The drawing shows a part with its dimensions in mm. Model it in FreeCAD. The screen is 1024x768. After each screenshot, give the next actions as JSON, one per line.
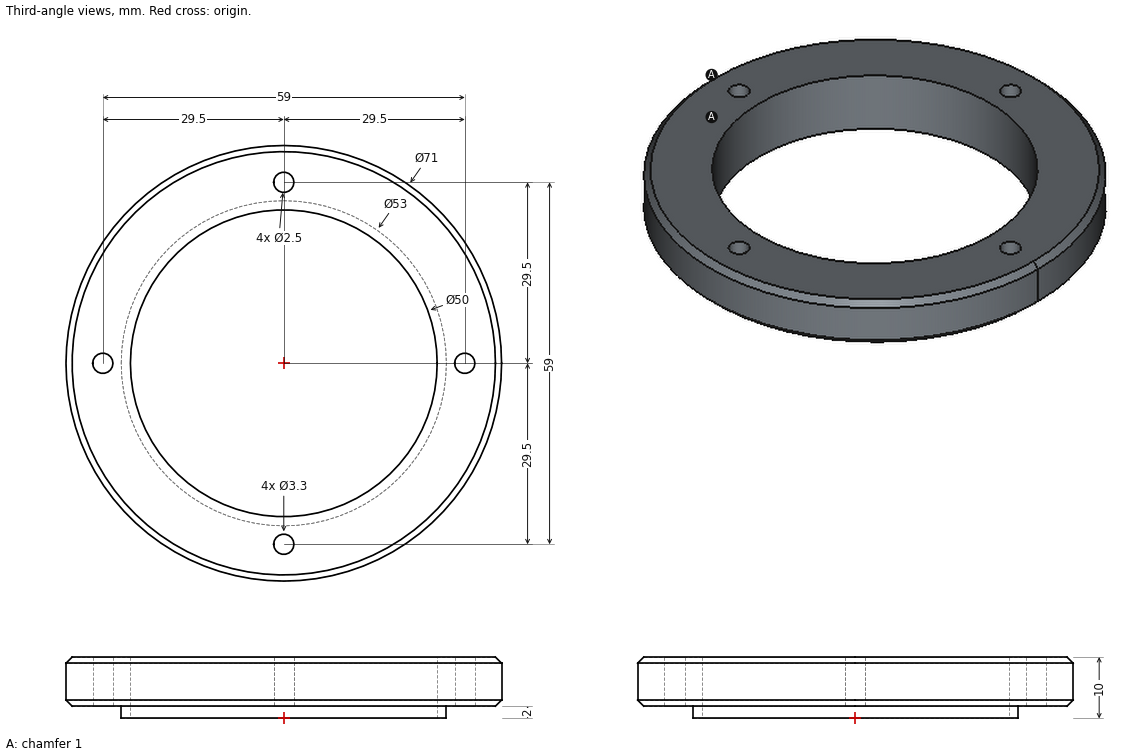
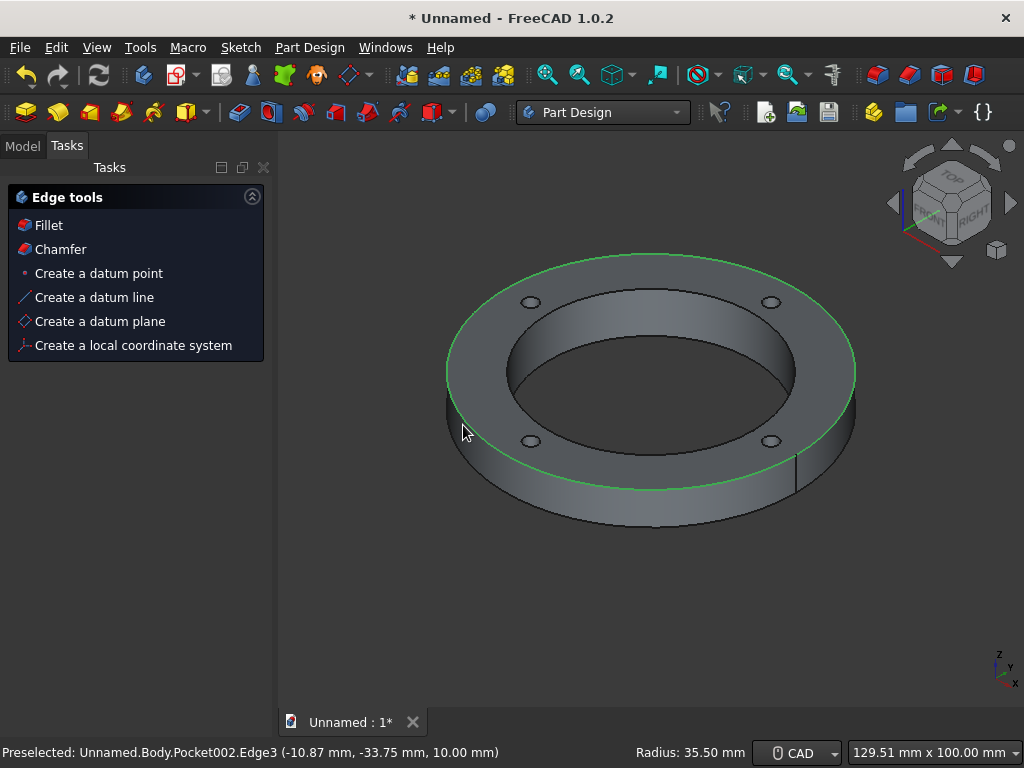
{"action": "key", "text": "1"}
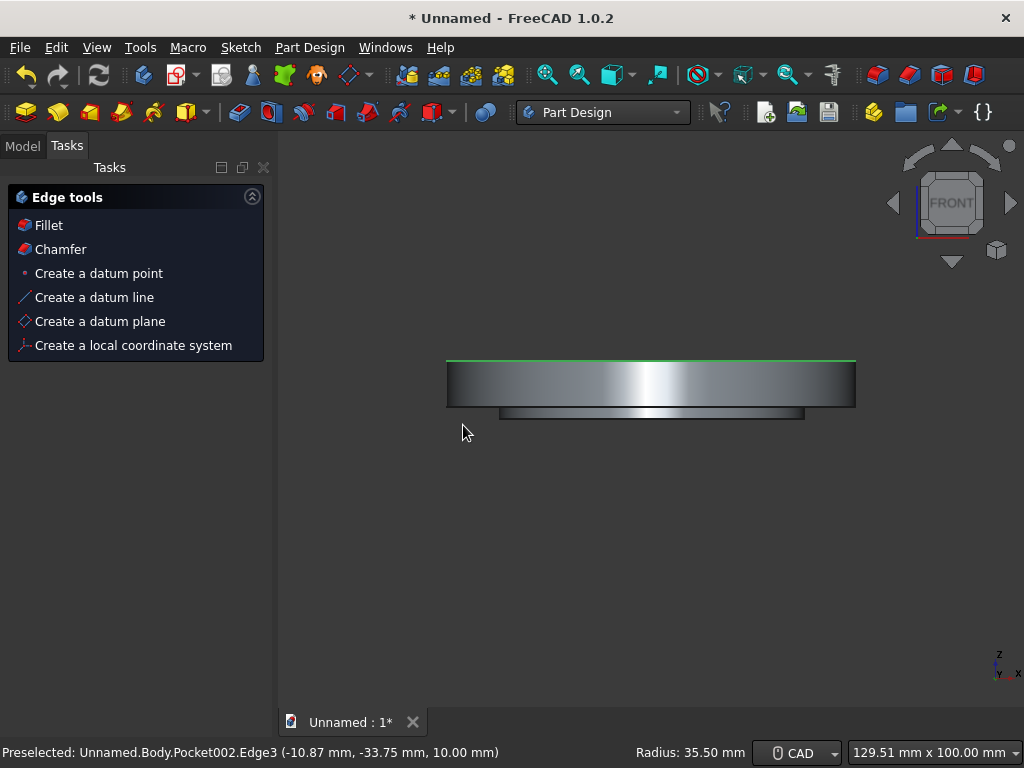
{"action": "left_click", "coordinate": [486, 406], "text": "ctrl"}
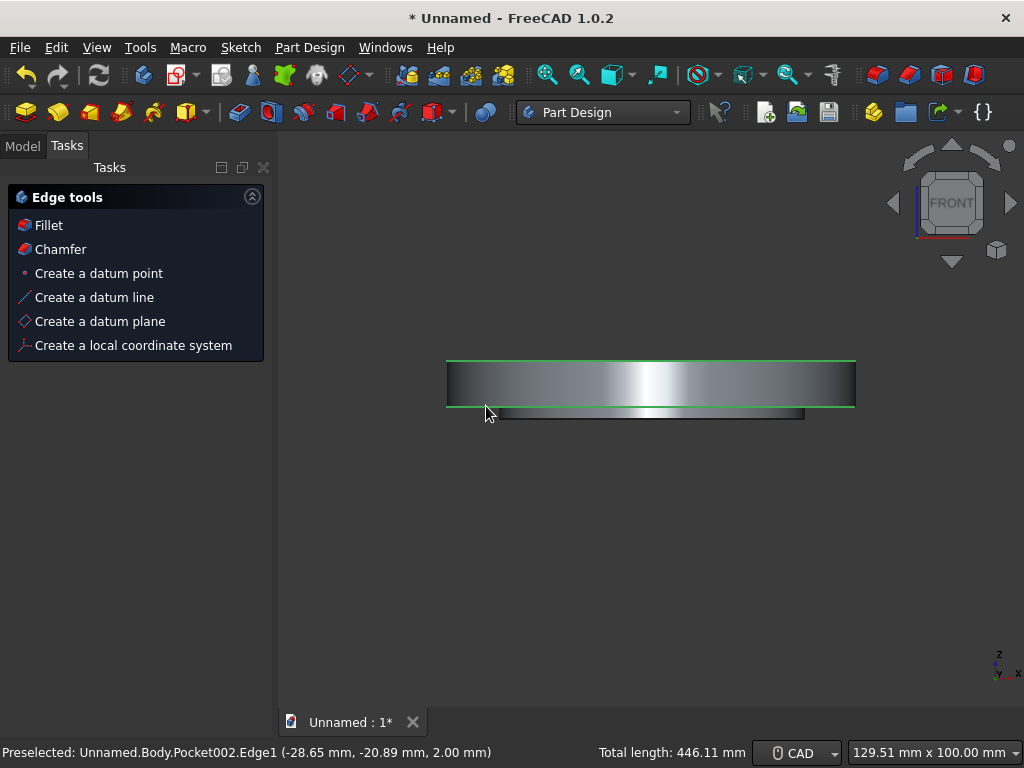
{"action": "left_click", "coordinate": [910, 76]}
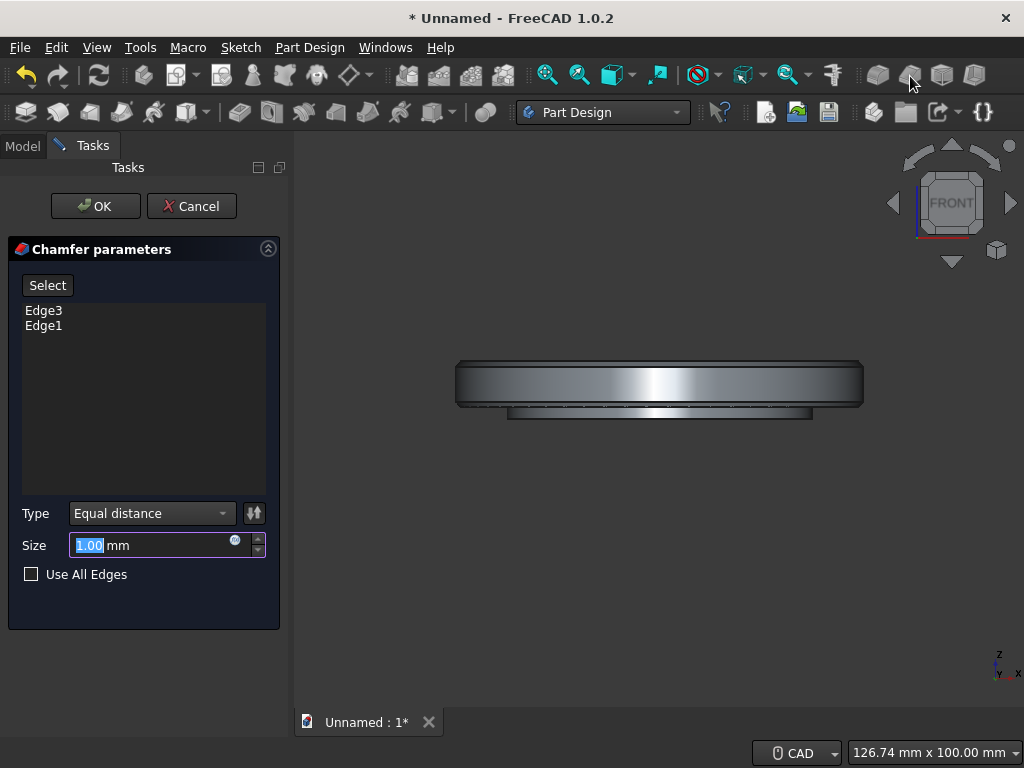
{"action": "type", "text": "1"}
{"action": "key", "text": "Tab"}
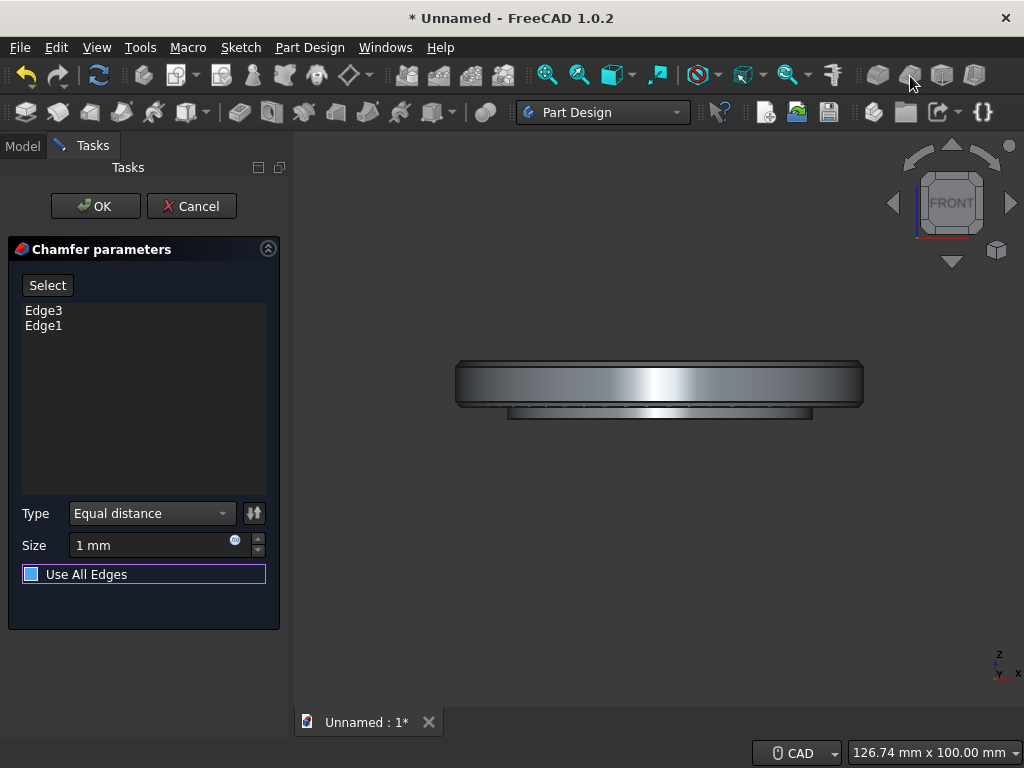
{"action": "left_click", "coordinate": [96, 206]}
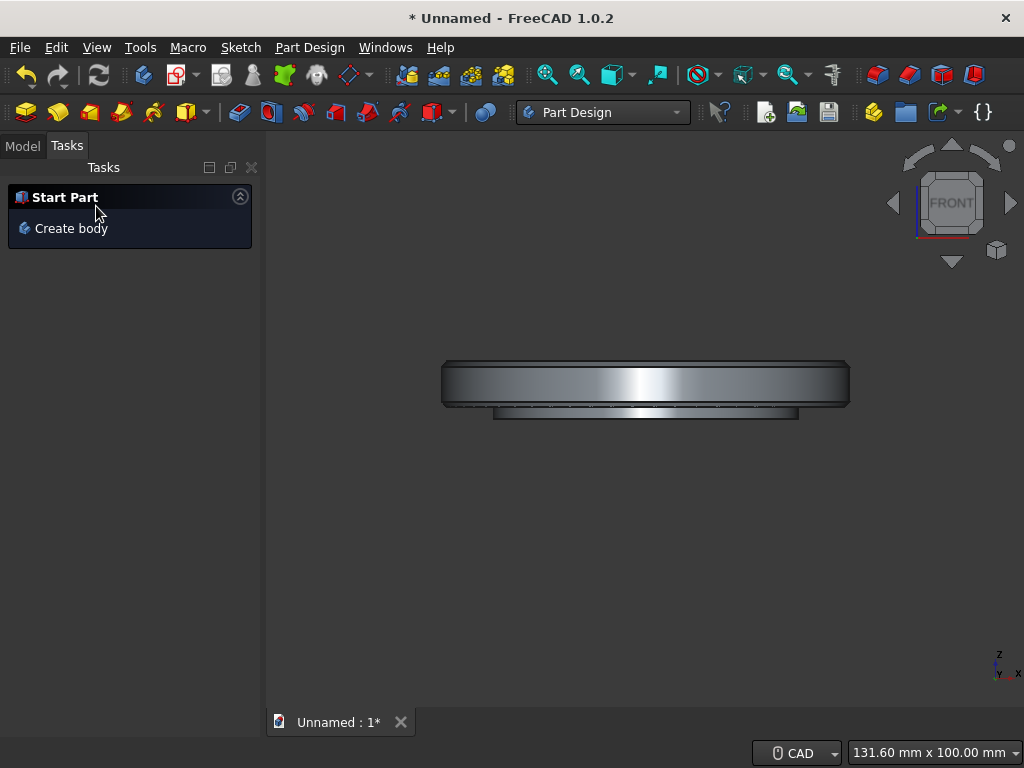
{"action": "key", "text": "0"}